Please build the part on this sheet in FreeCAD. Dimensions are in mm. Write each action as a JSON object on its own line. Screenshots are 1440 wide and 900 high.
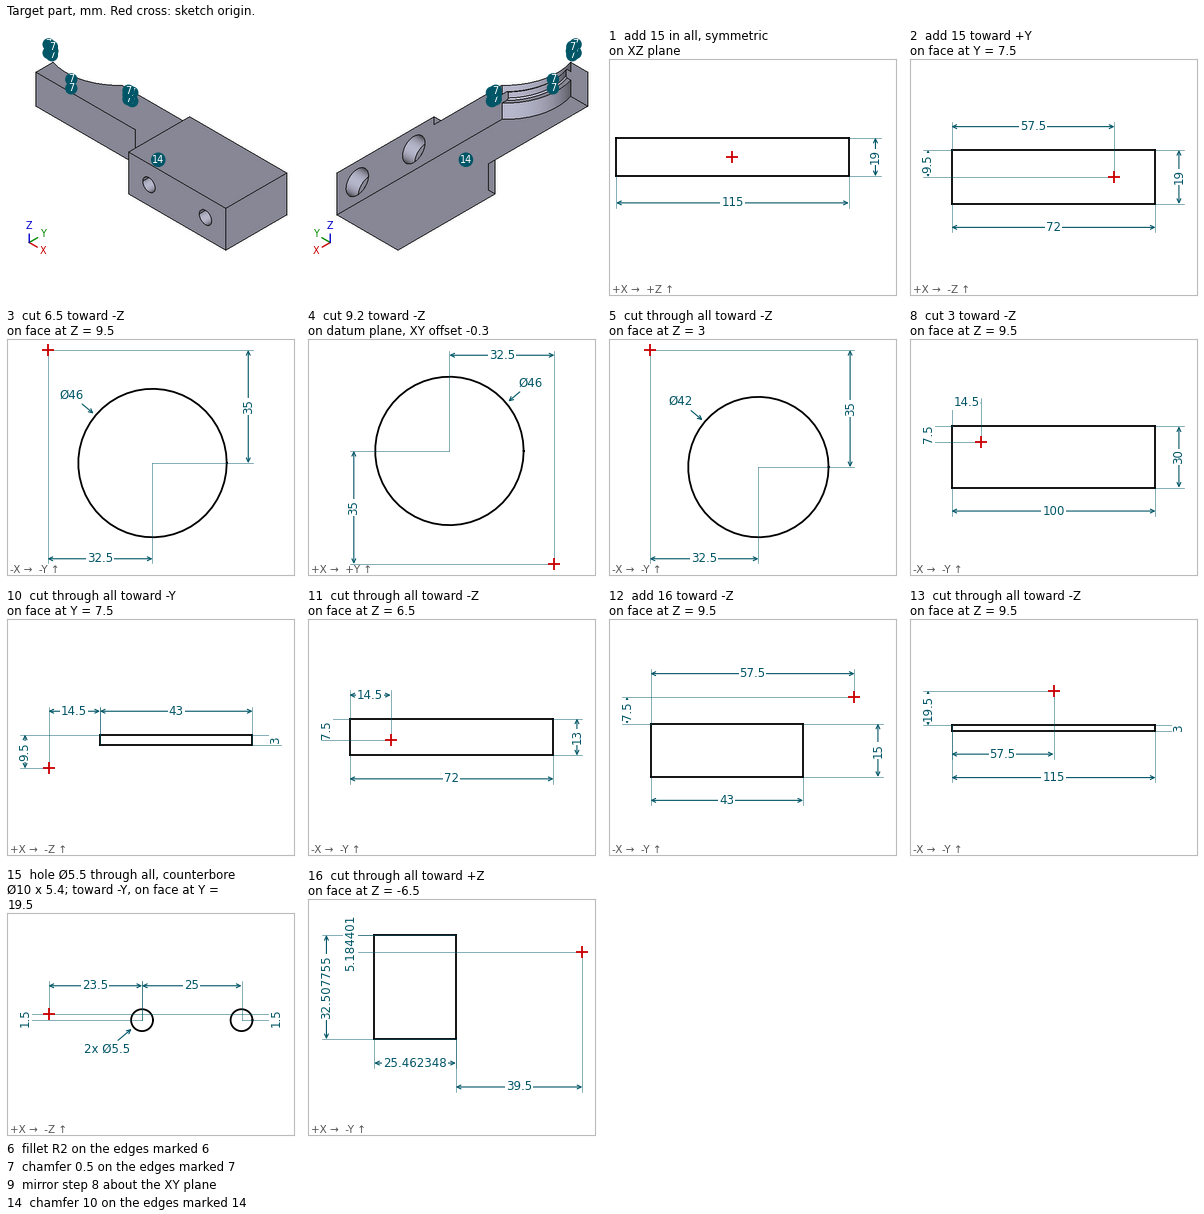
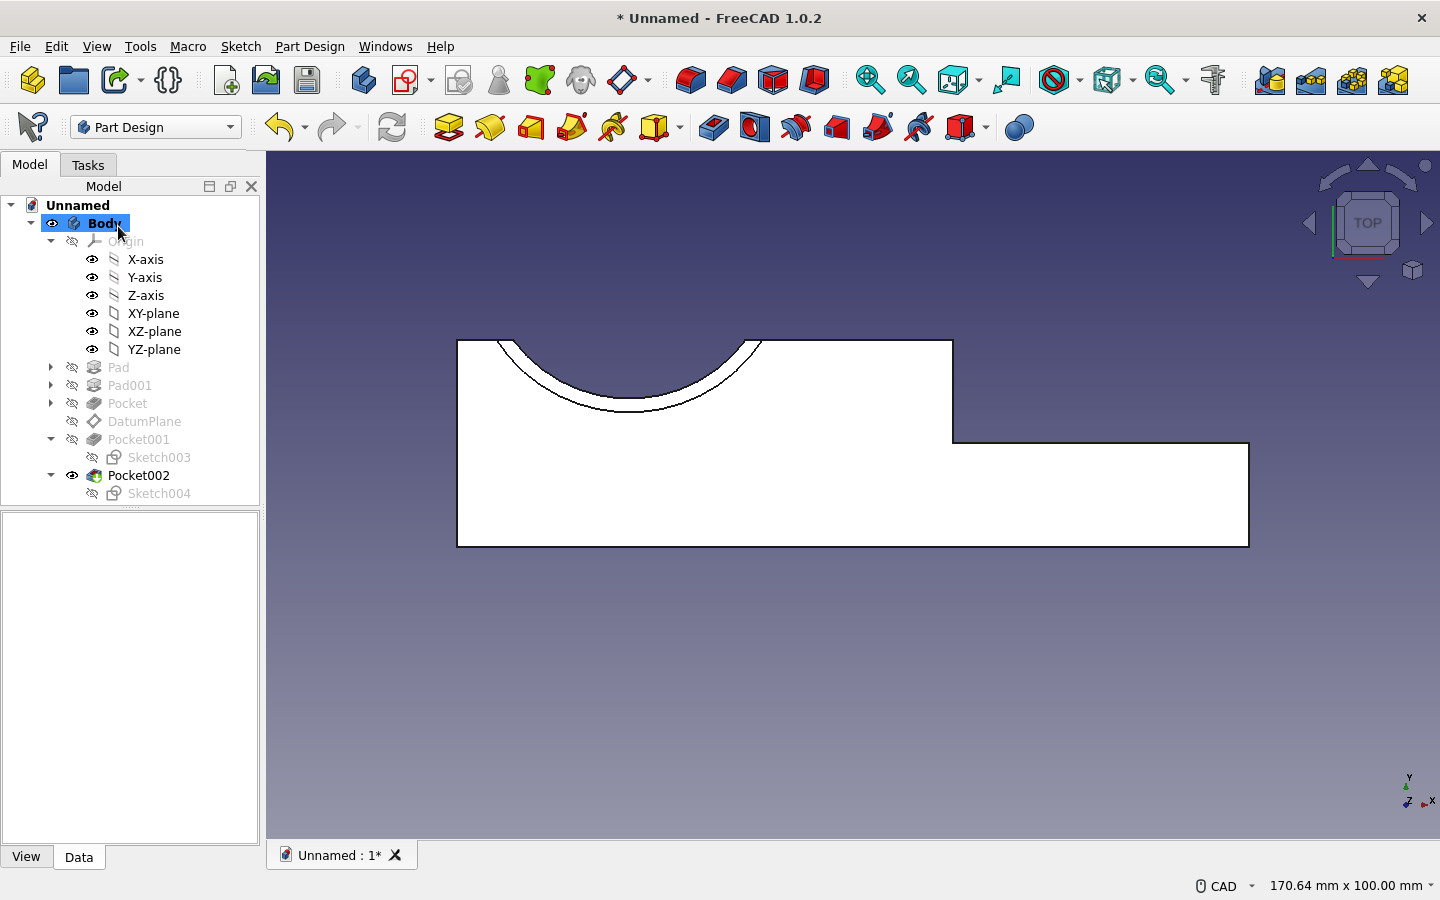
{"action": "key", "text": "1"}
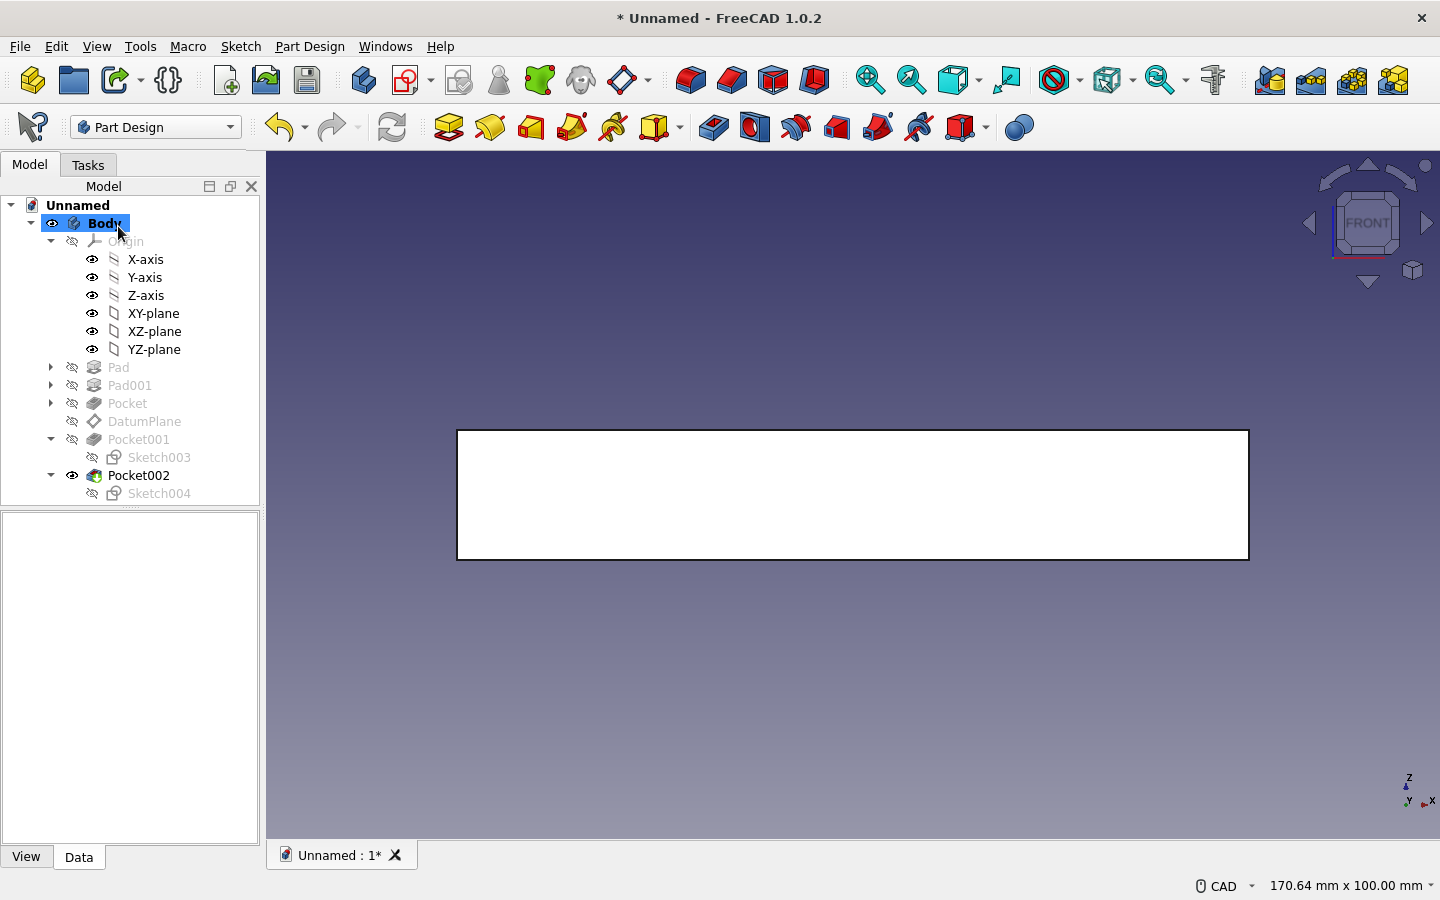
{"action": "key", "text": "3"}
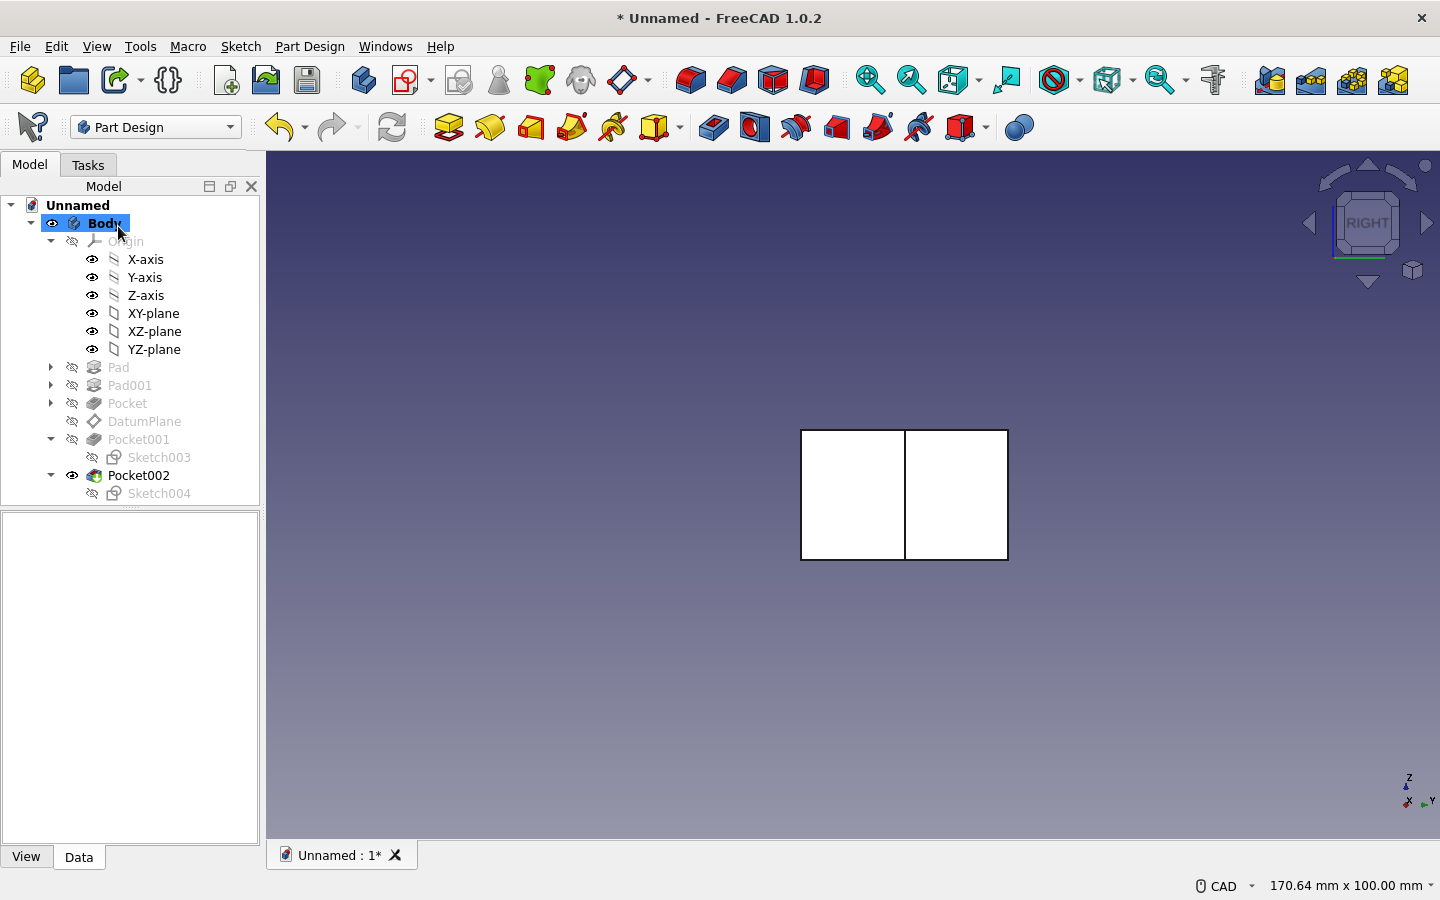
{"action": "left_click", "coordinate": [871, 80]}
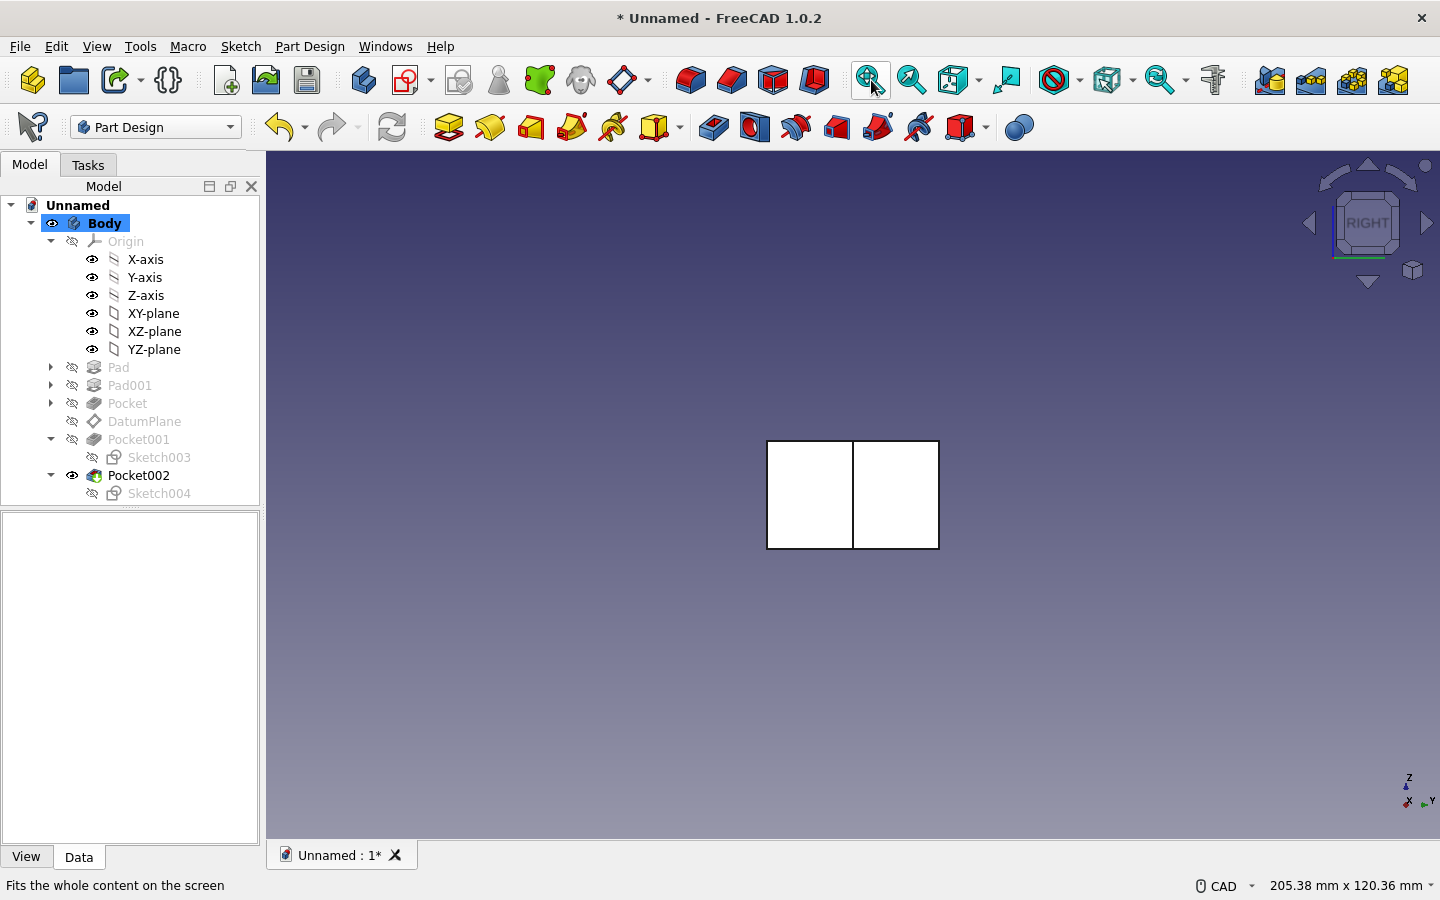
{"action": "scroll", "coordinate": [939, 486], "scroll_direction": "up", "scroll_amount": 4}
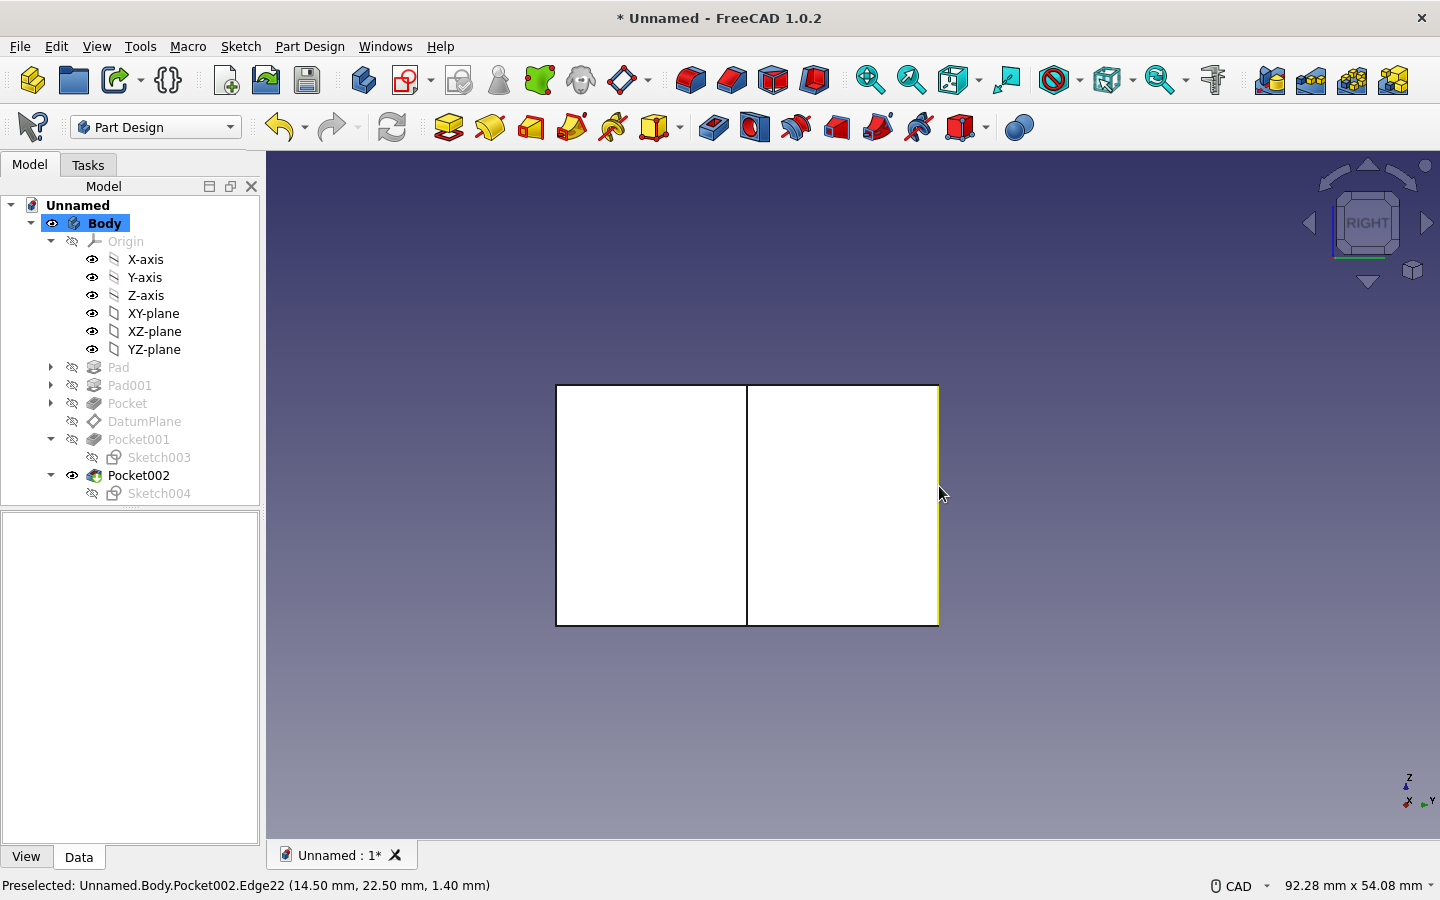
{"action": "left_click", "coordinate": [871, 80]}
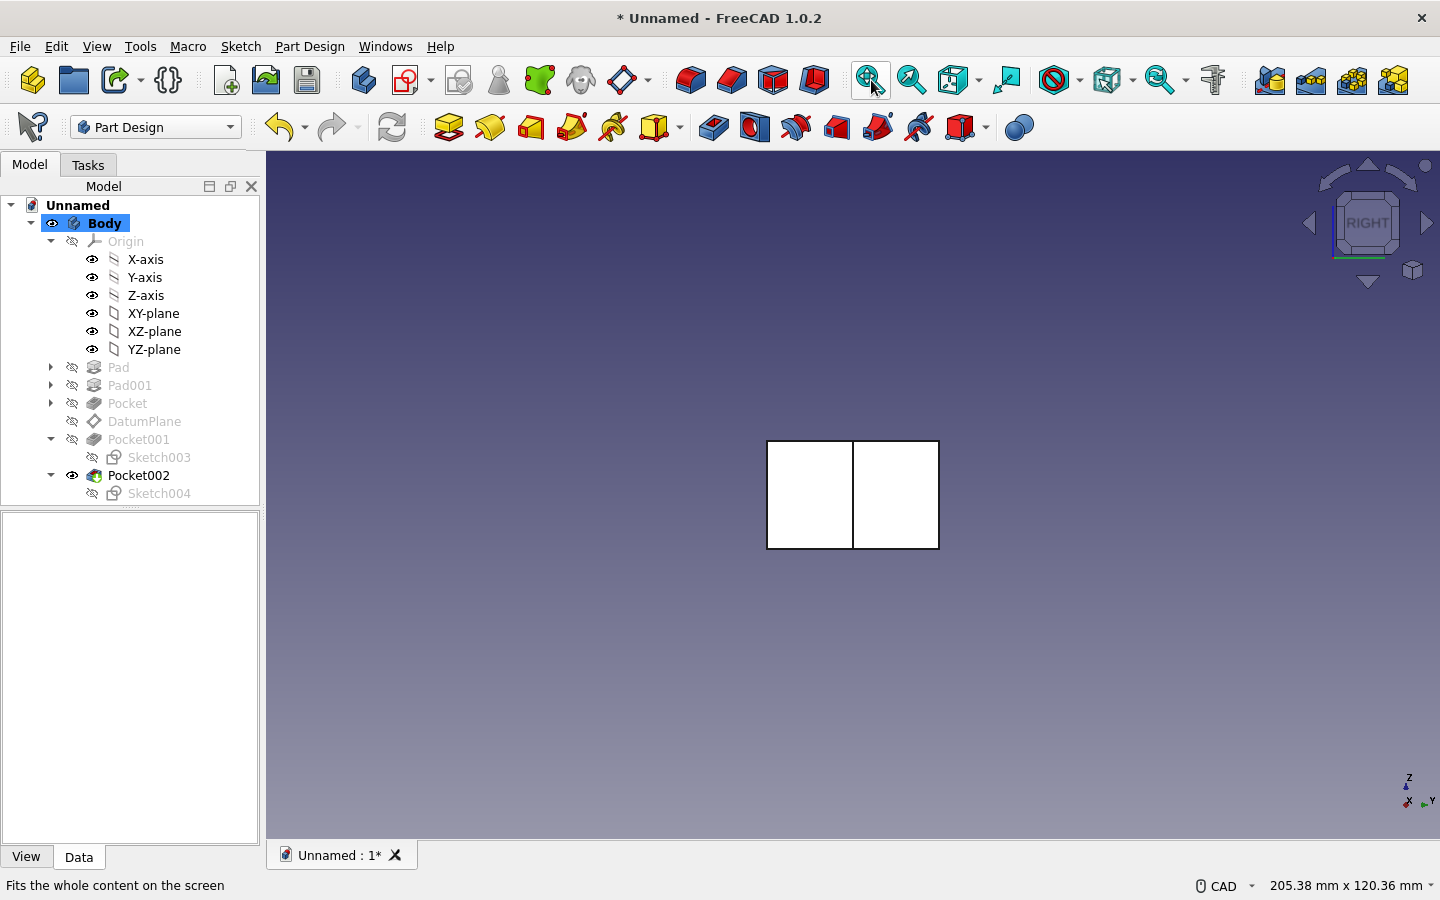
{"action": "key", "text": "5"}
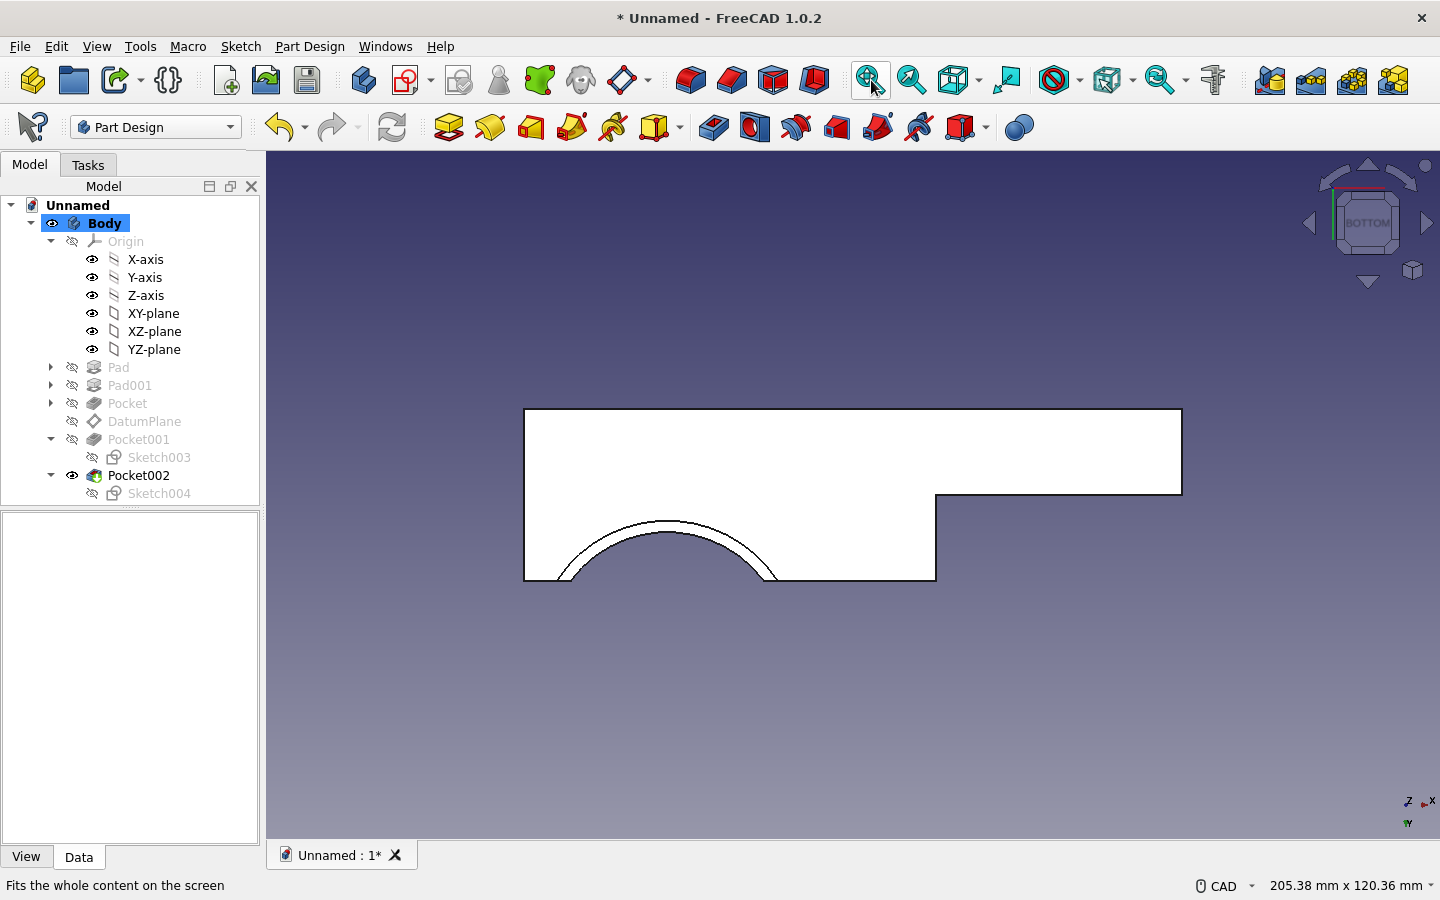
{"action": "scroll", "coordinate": [571, 580], "scroll_direction": "up", "scroll_amount": 4}